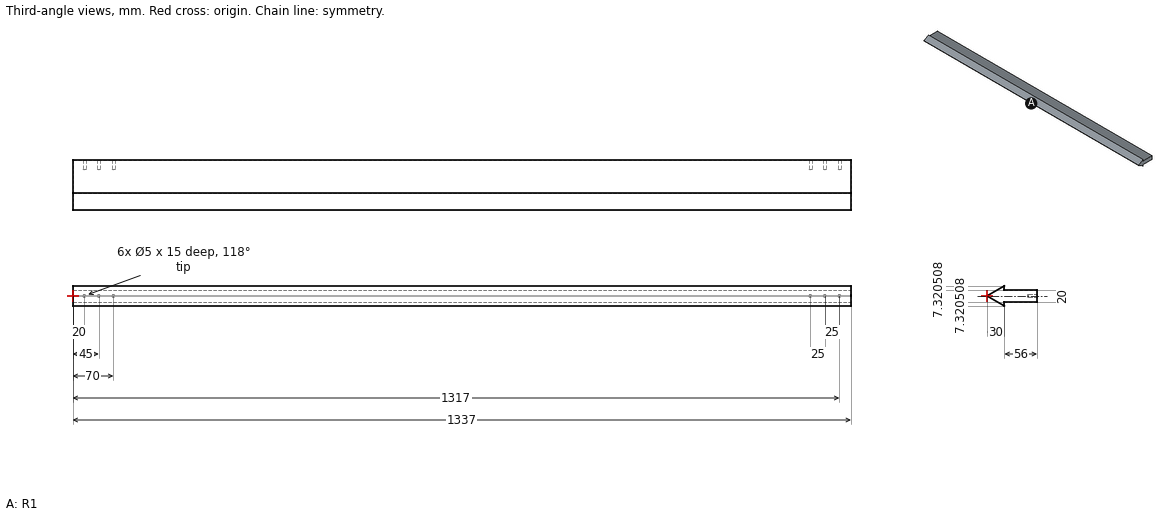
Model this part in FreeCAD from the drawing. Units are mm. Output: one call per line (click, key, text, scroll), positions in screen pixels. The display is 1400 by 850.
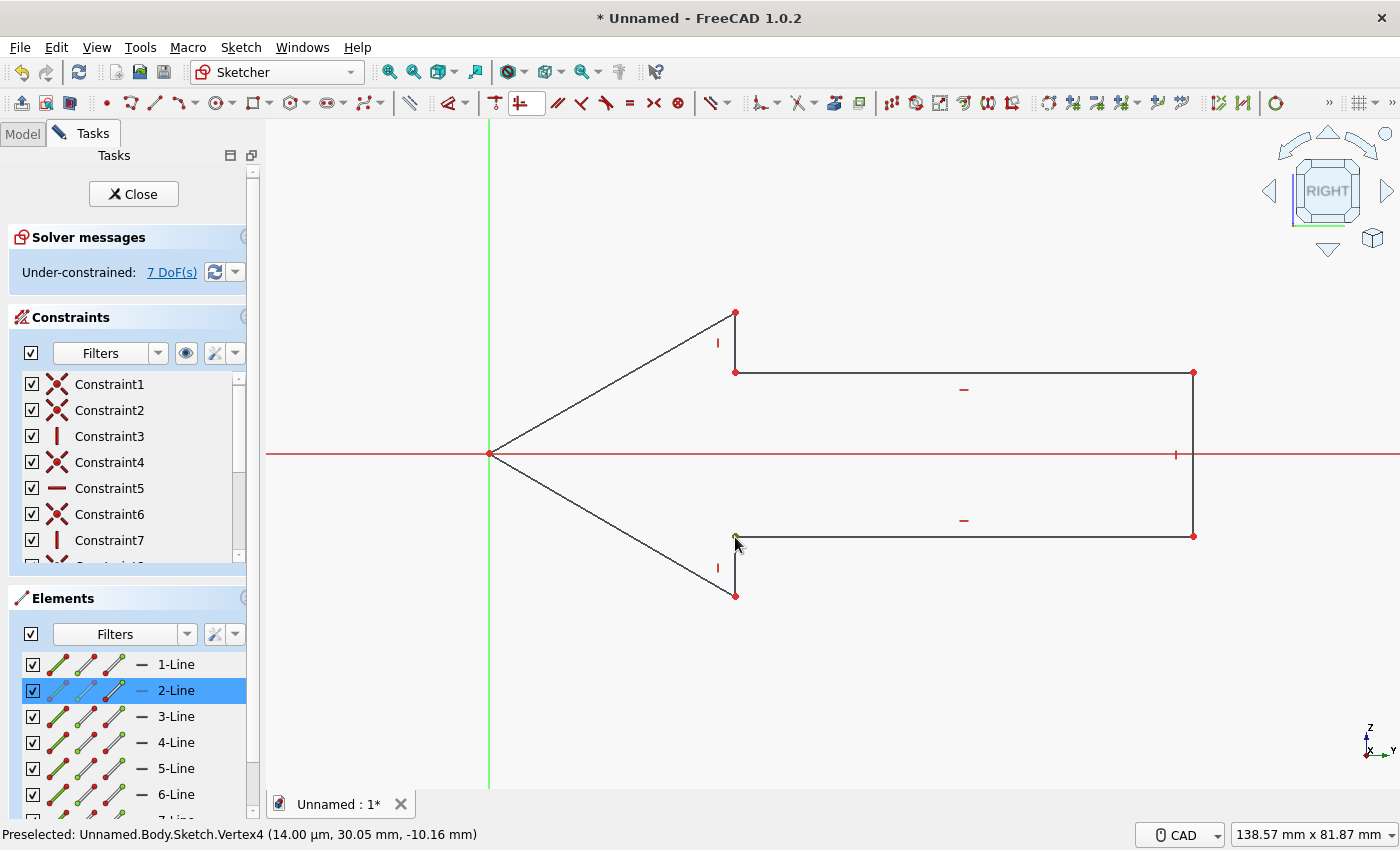
click(735, 373)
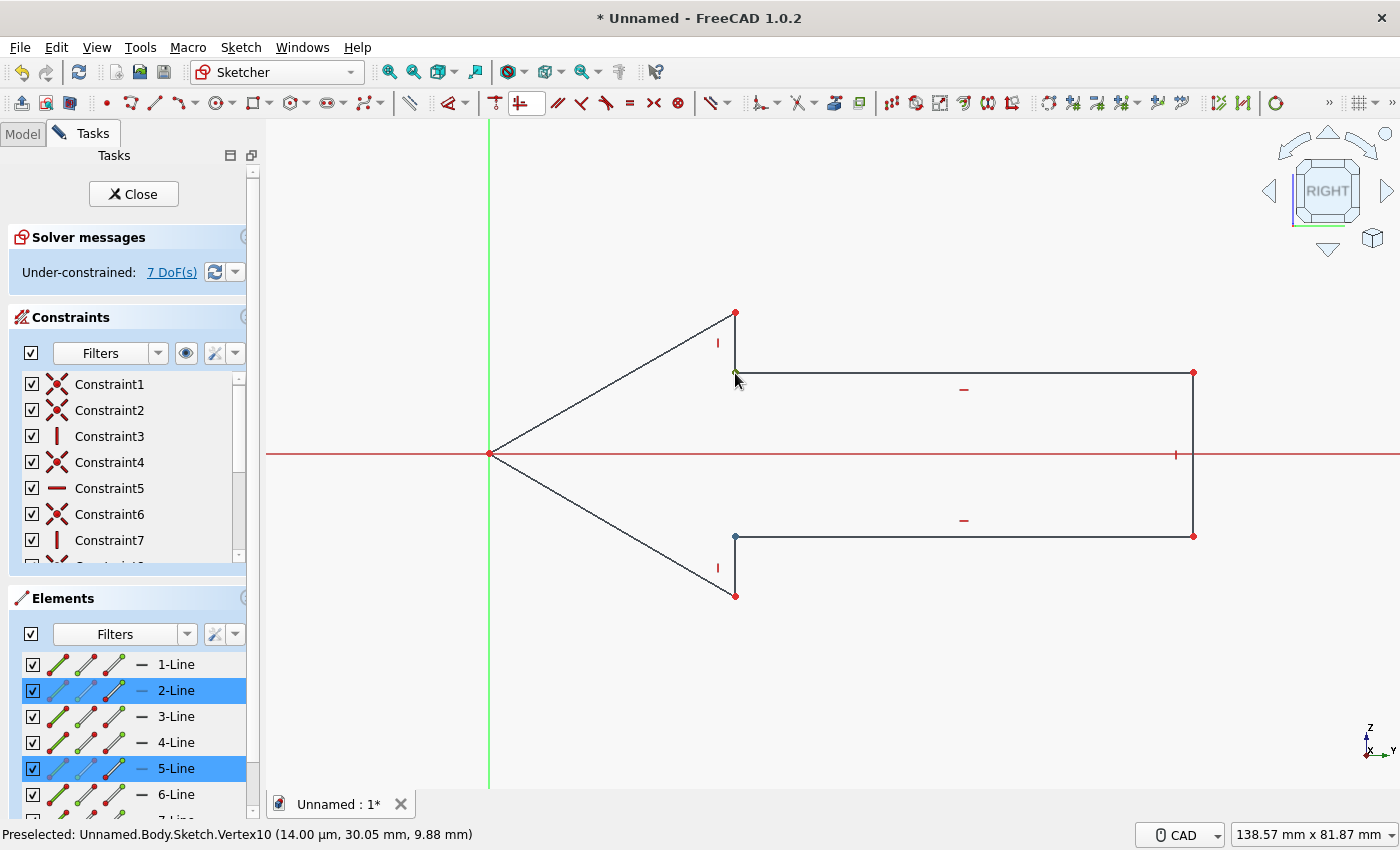
click(361, 454)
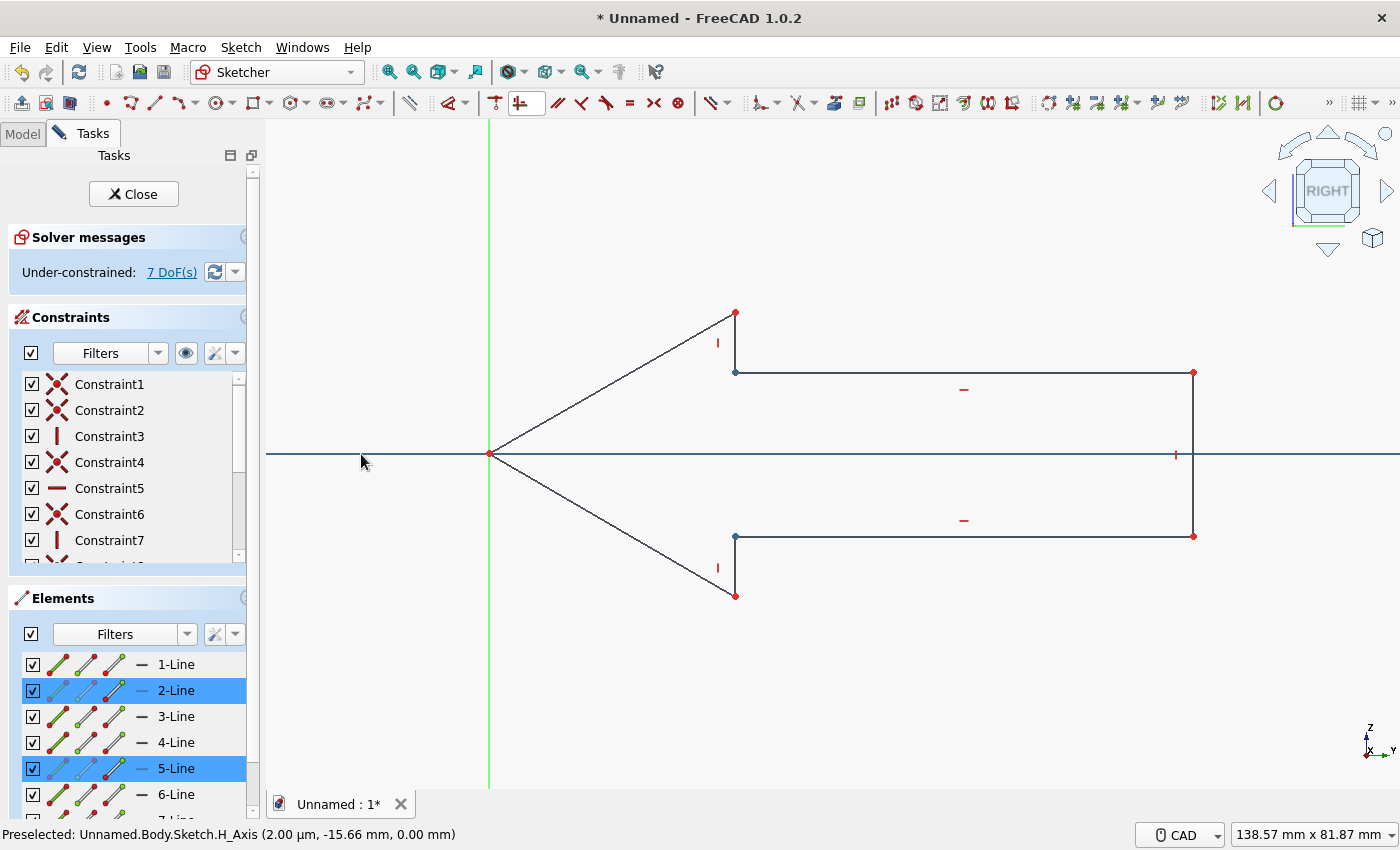
click(654, 104)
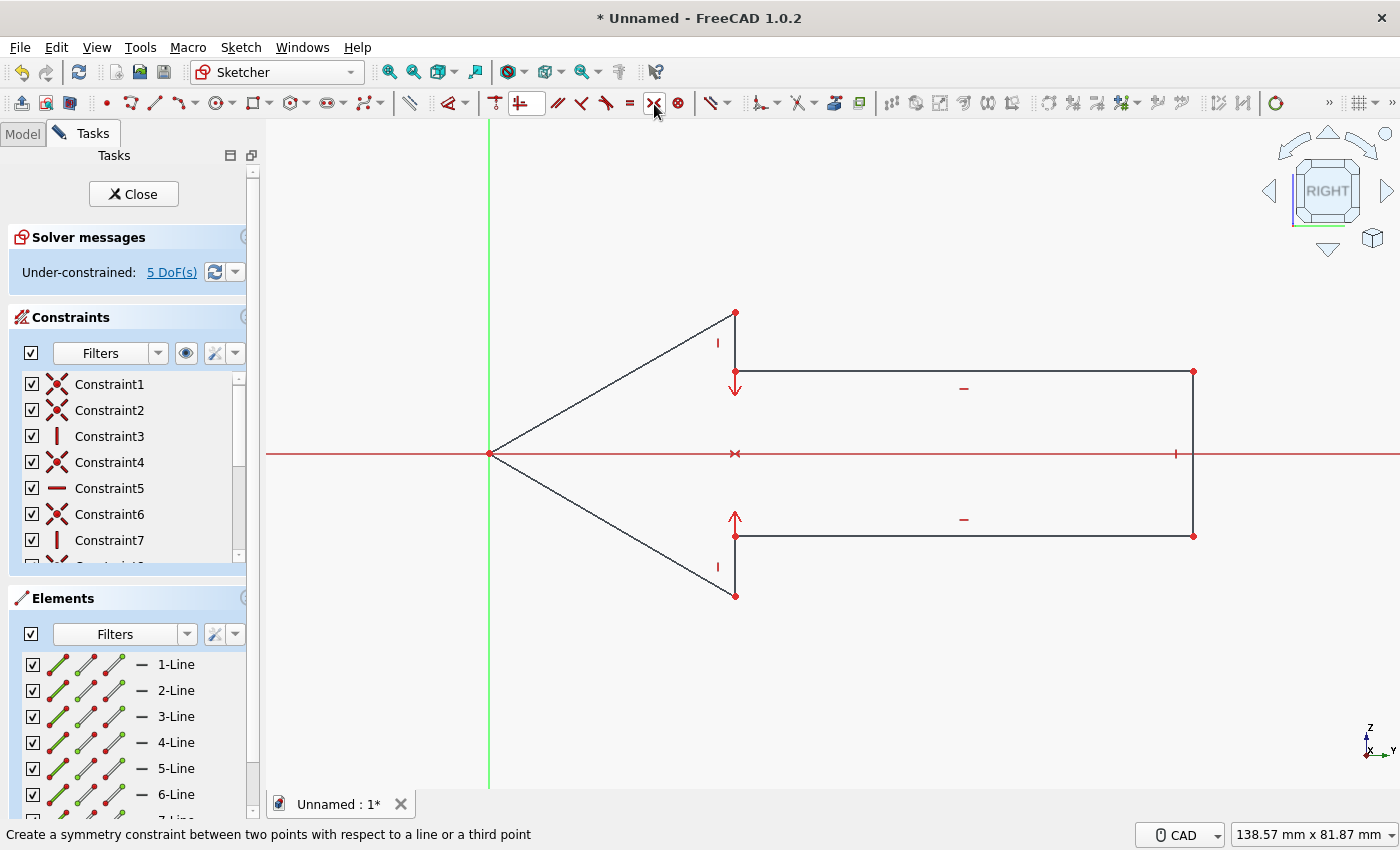
click(448, 104)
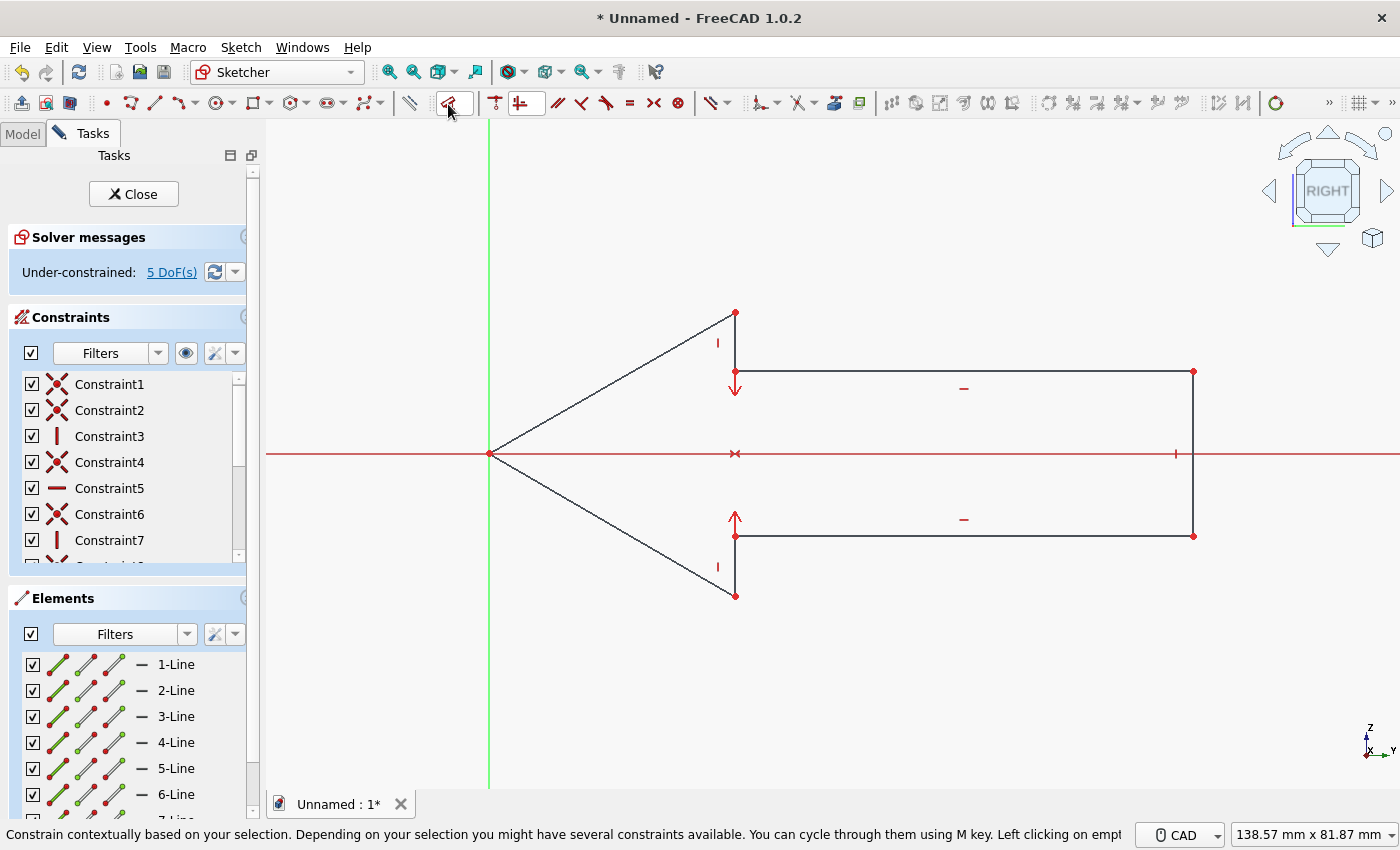
click(872, 536)
click(964, 570)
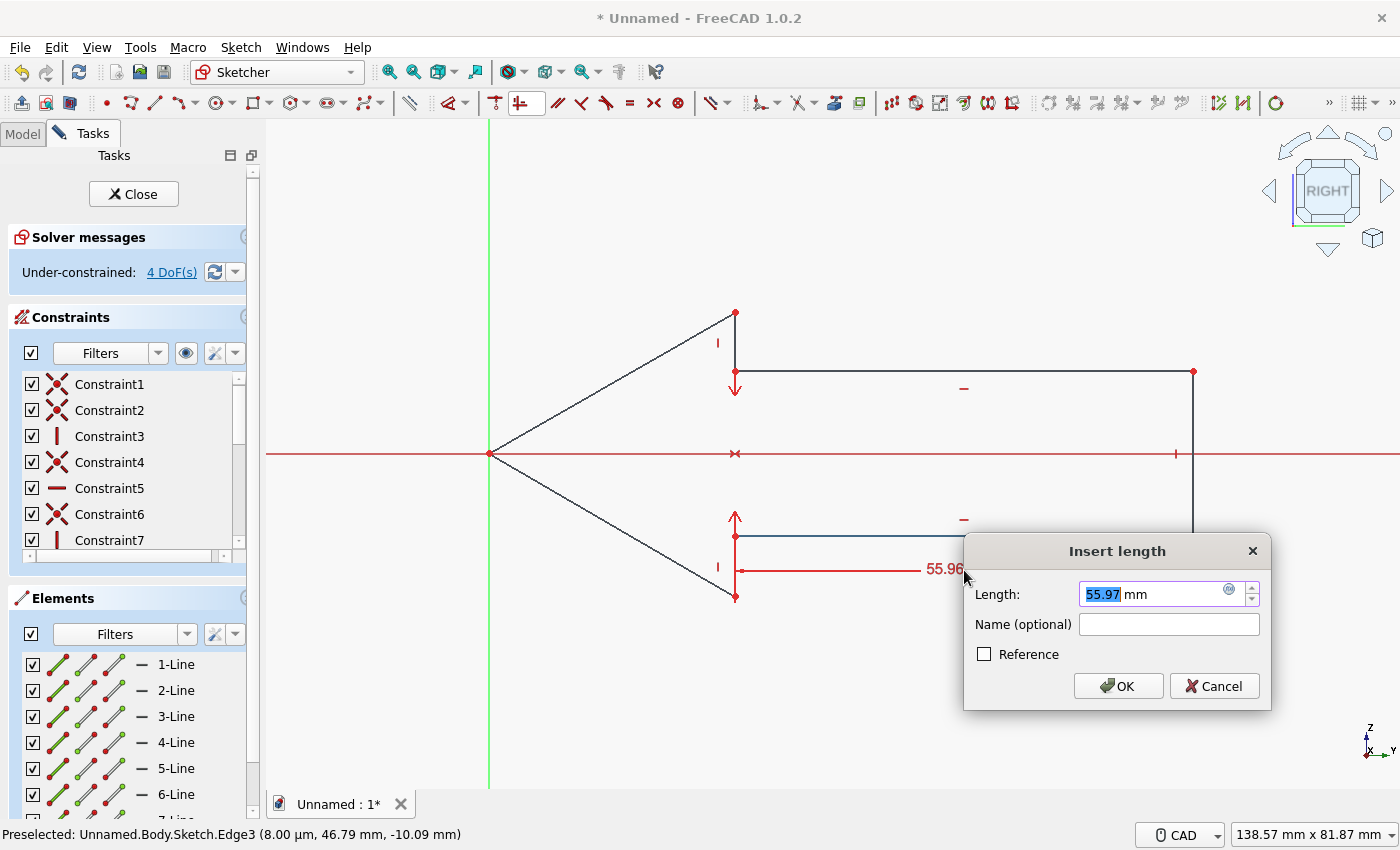
text(56)
key(Return)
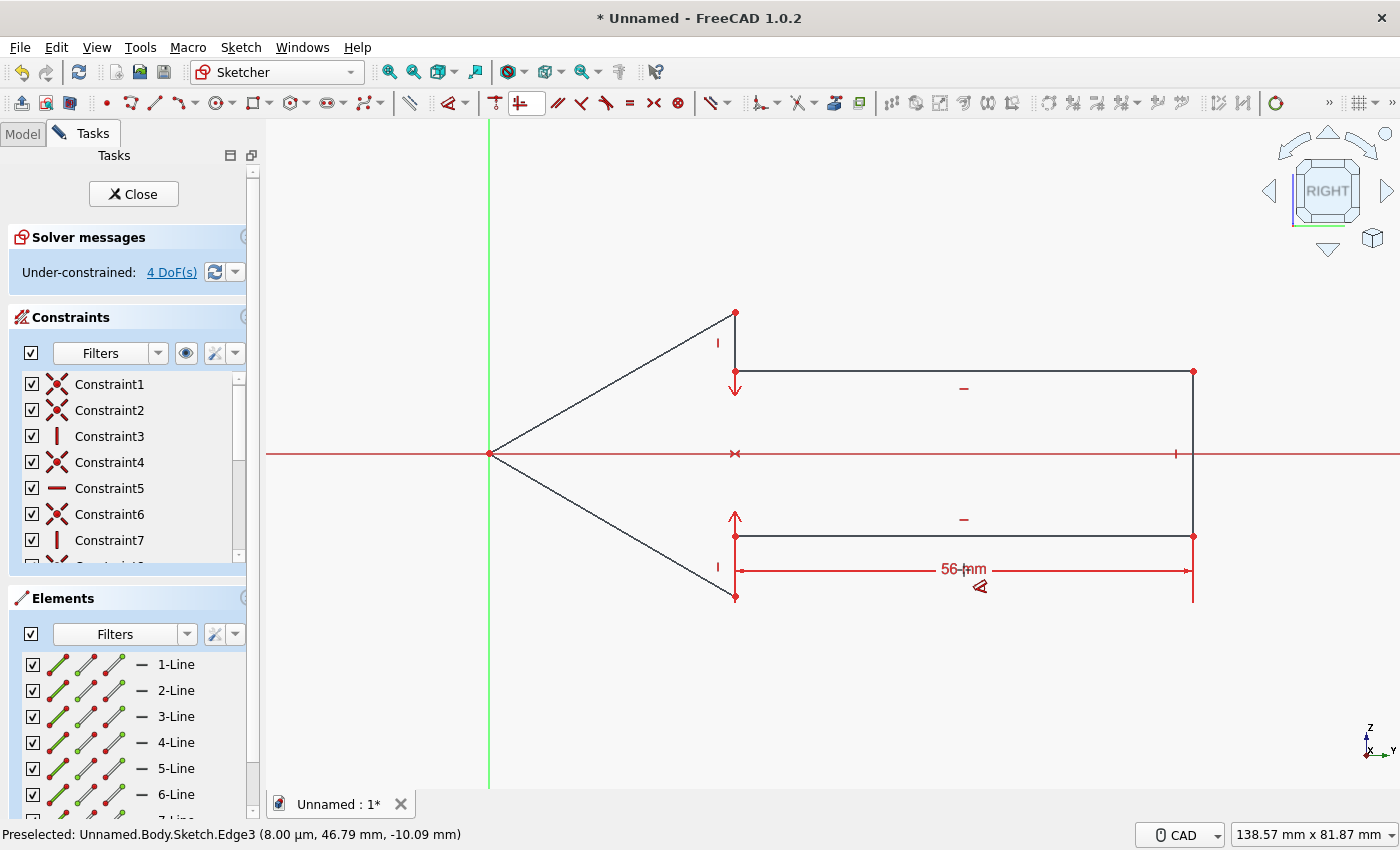
click(1193, 487)
click(1227, 416)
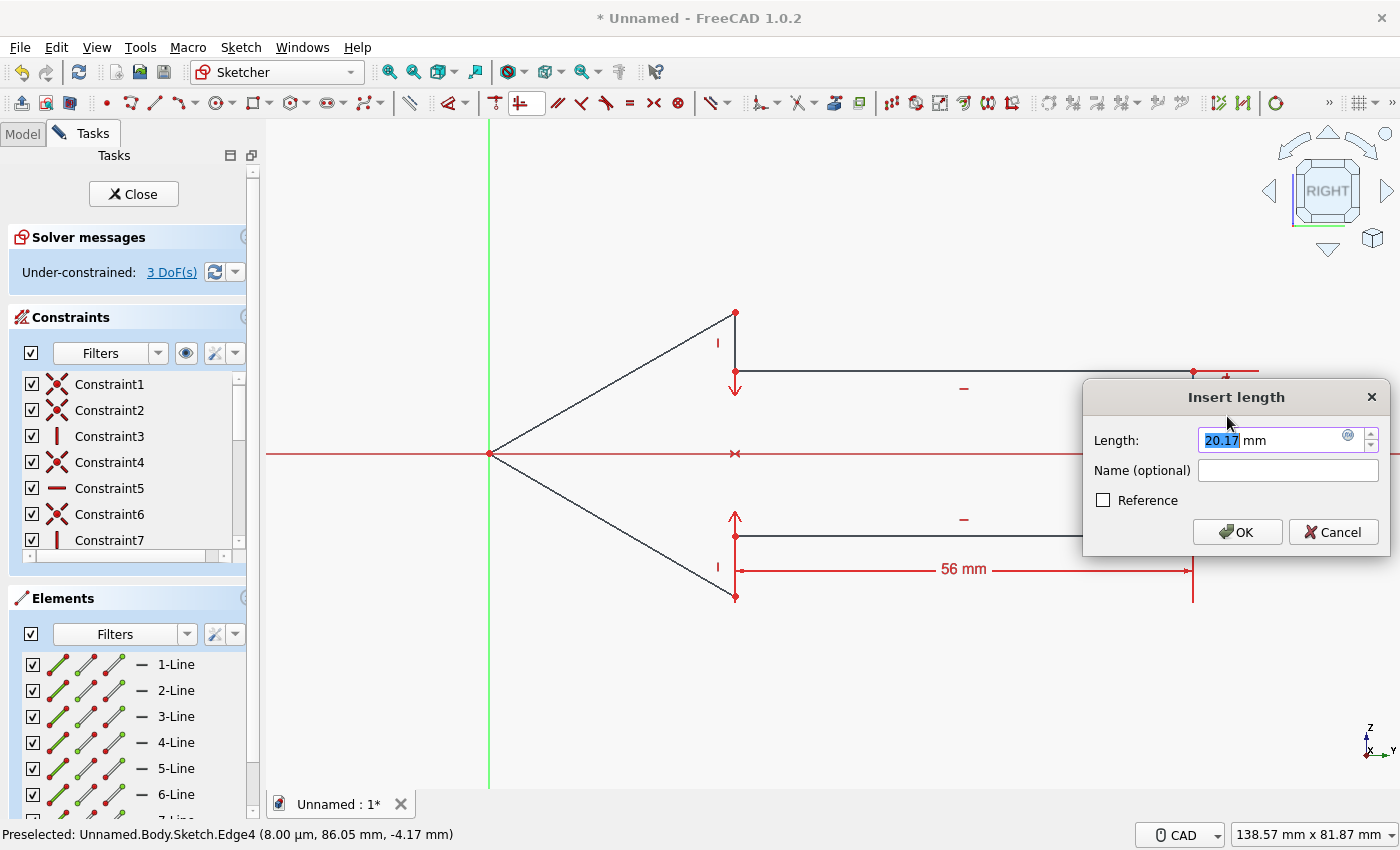
text(20)
key(Return)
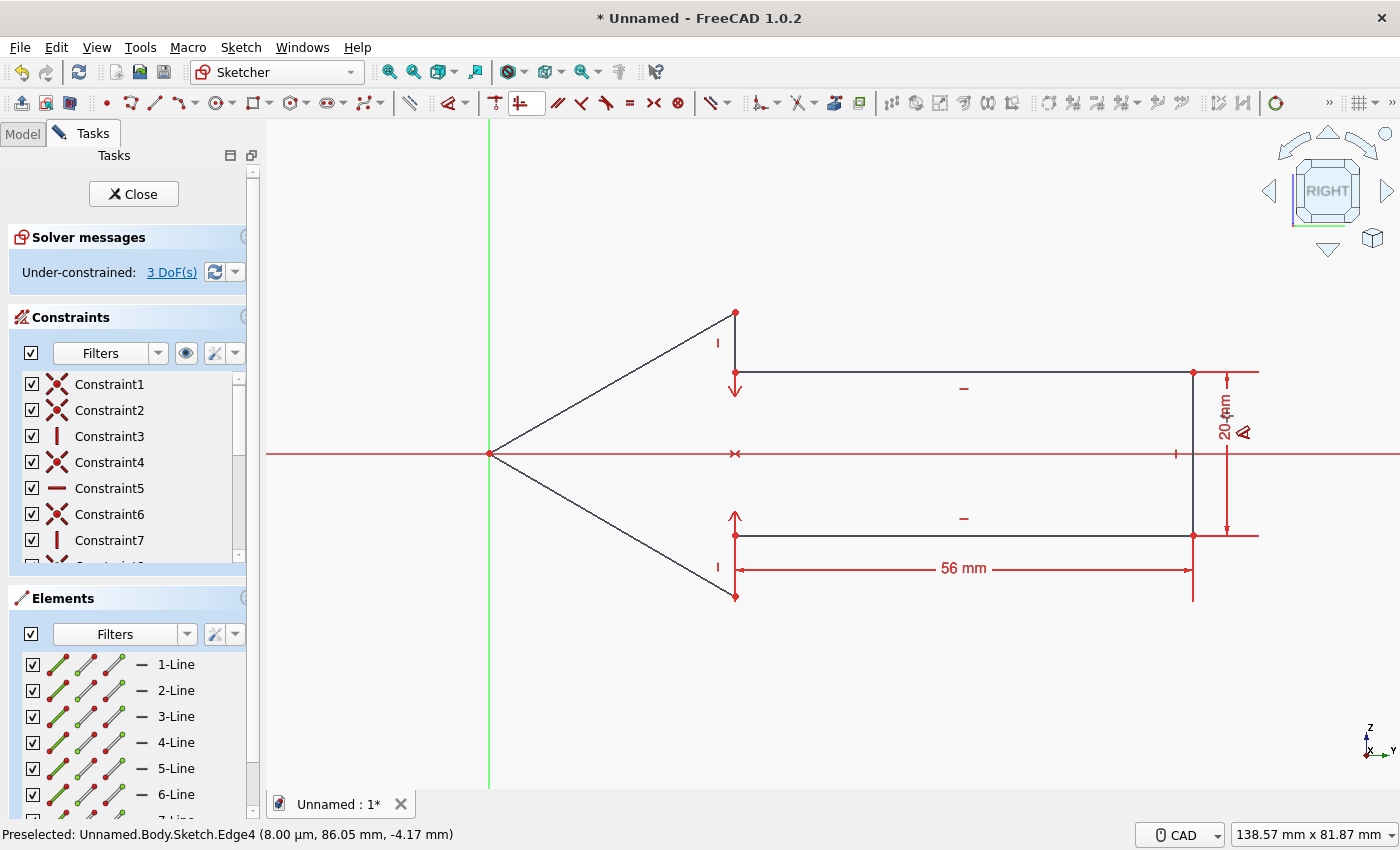
click(735, 597)
click(612, 631)